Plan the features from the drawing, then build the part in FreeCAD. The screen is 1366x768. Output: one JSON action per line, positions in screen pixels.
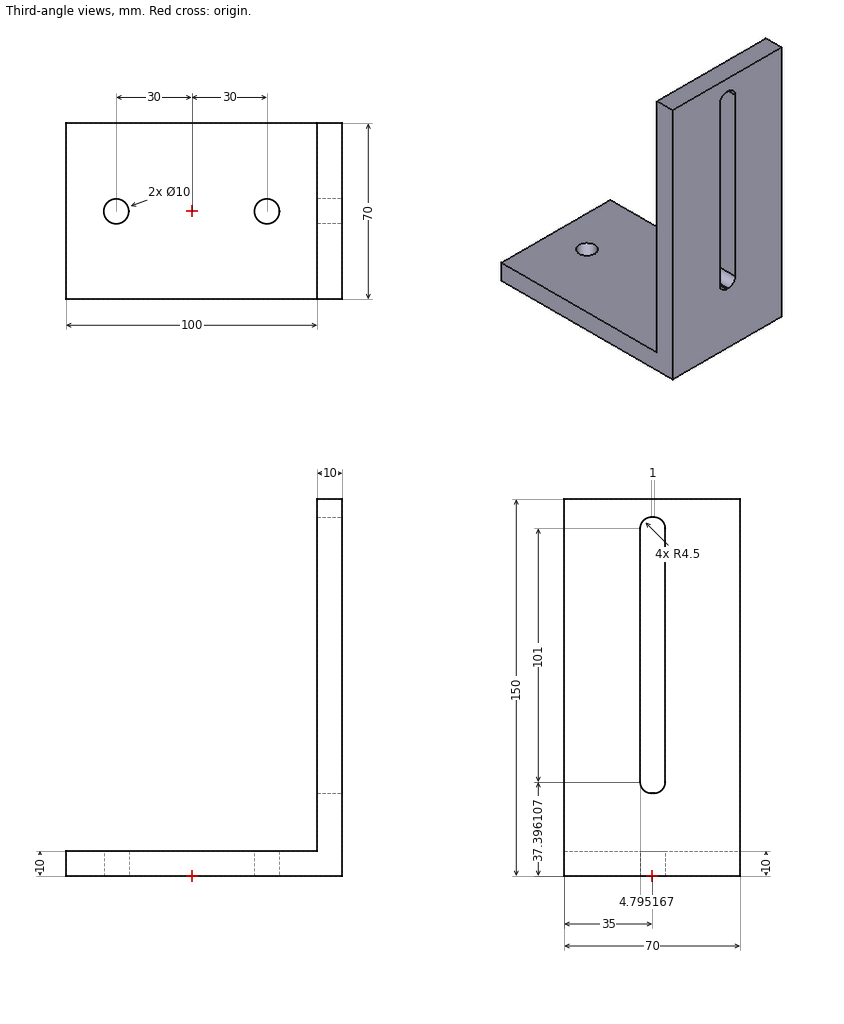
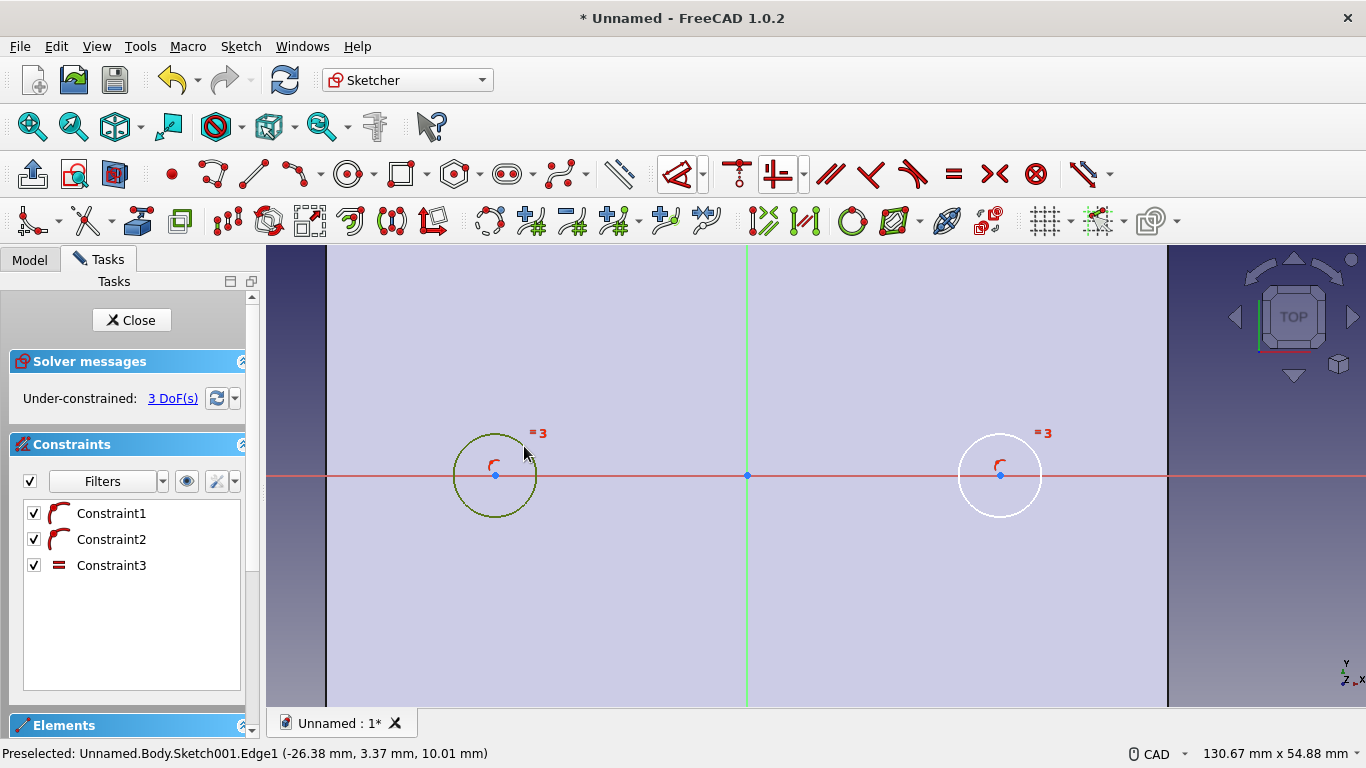
{"action": "left_click", "coordinate": [702, 174]}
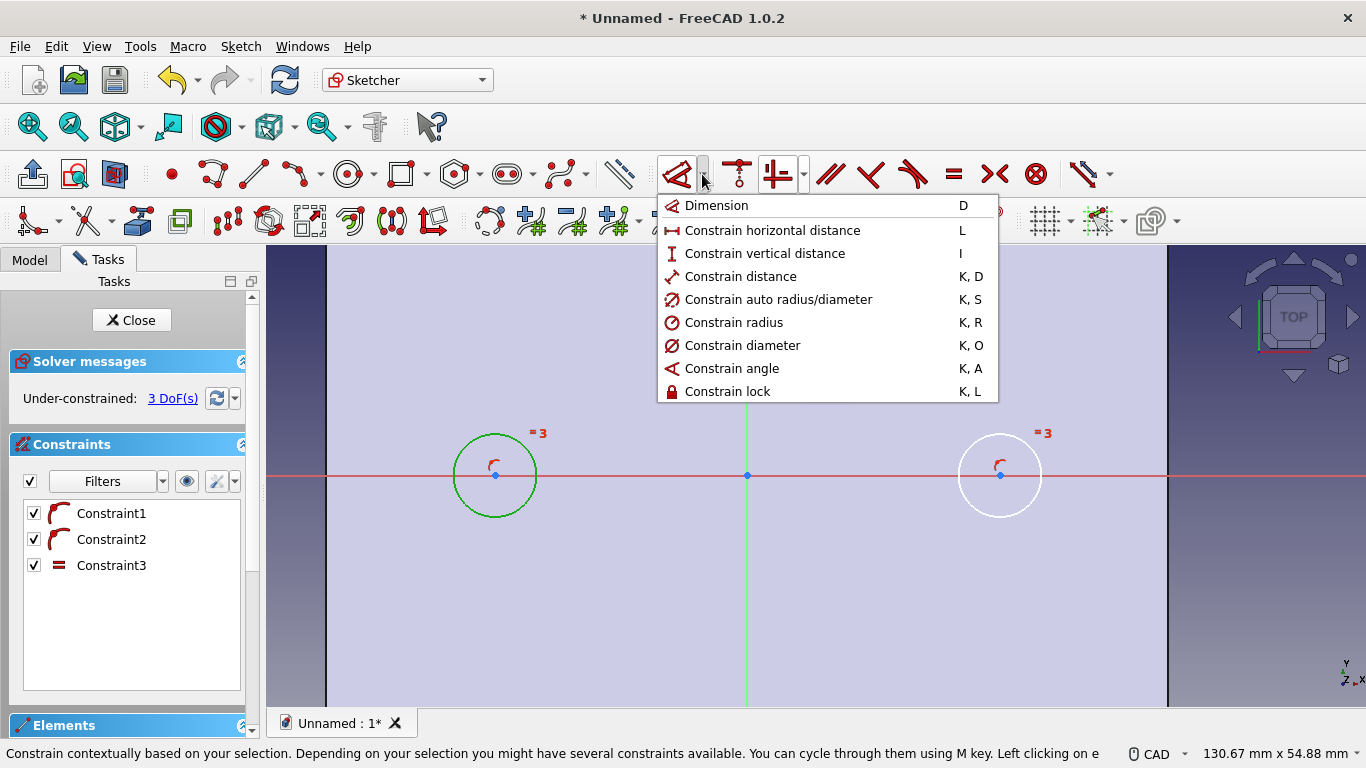
{"action": "left_click", "coordinate": [828, 346]}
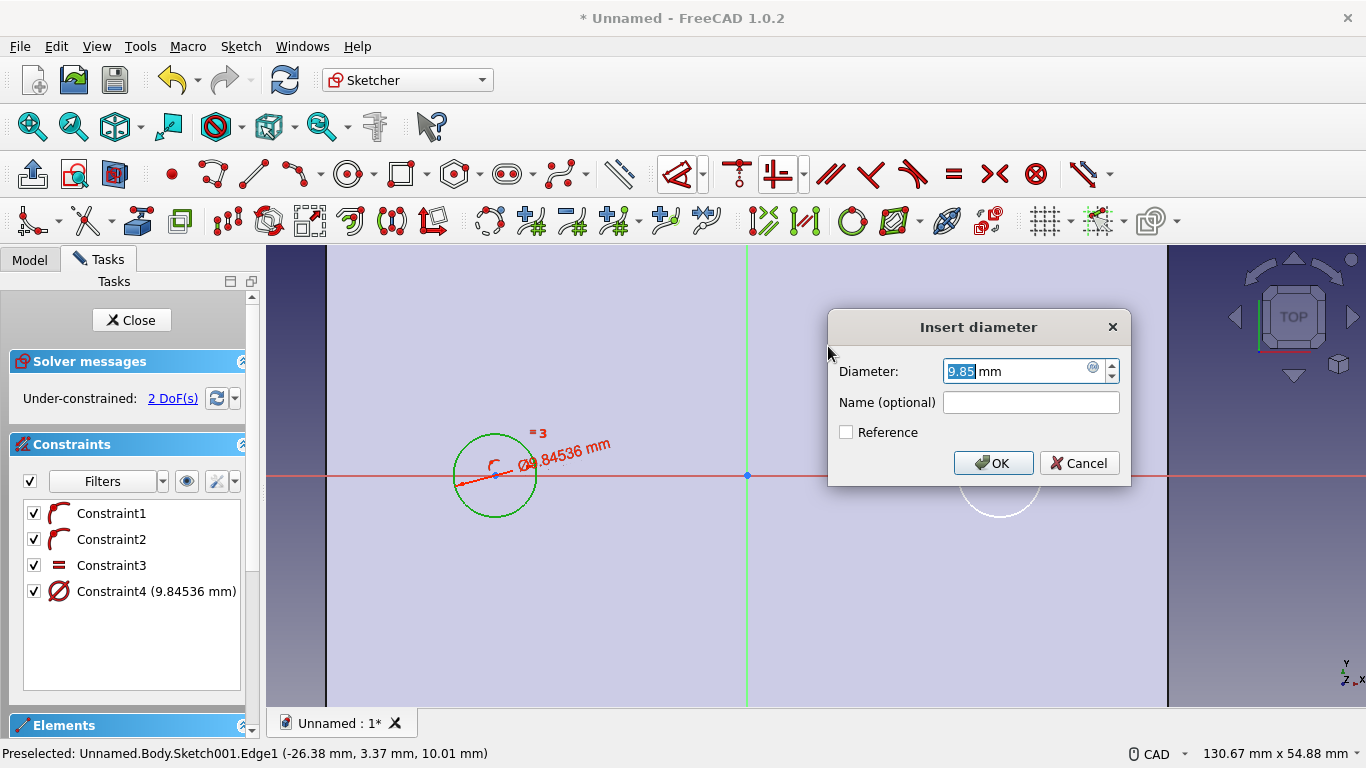
{"action": "type", "text": "10"}
{"action": "key", "text": "Return"}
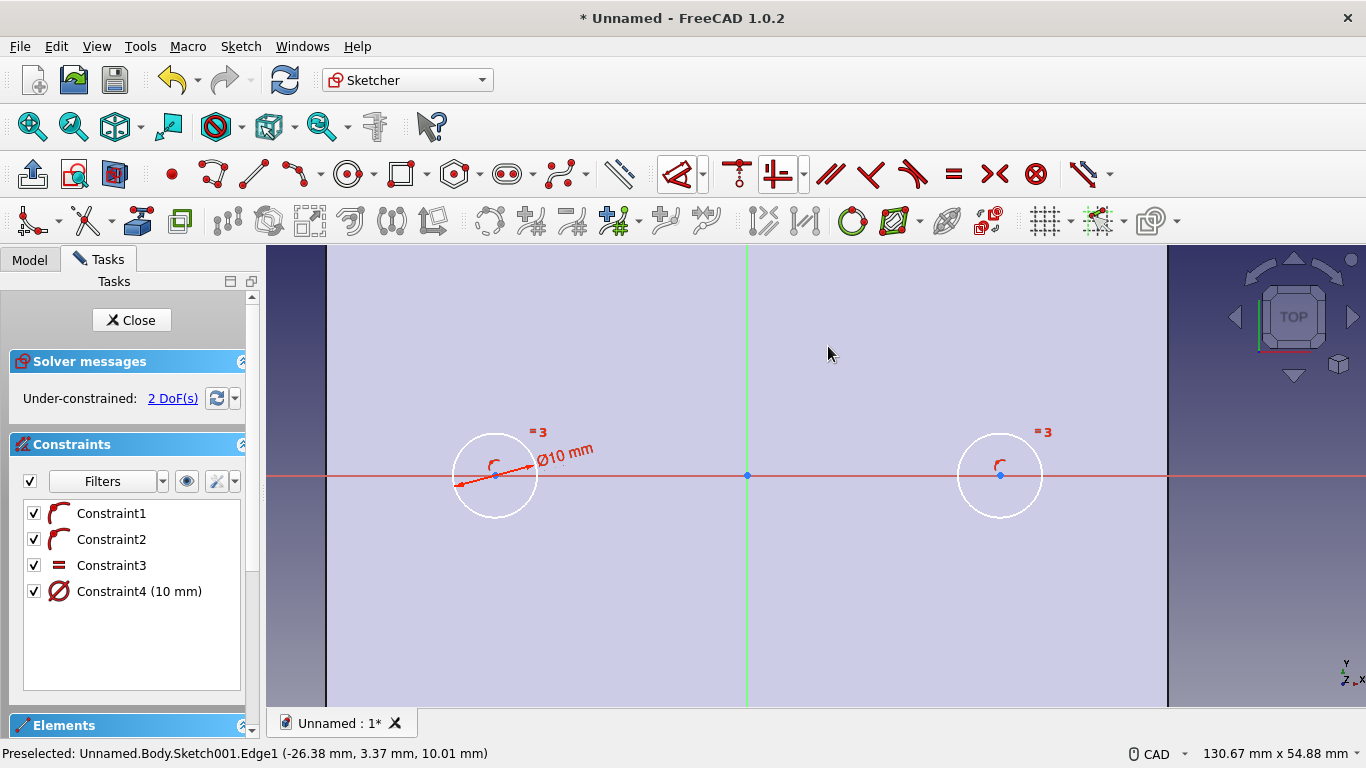
{"action": "left_click", "coordinate": [495, 476]}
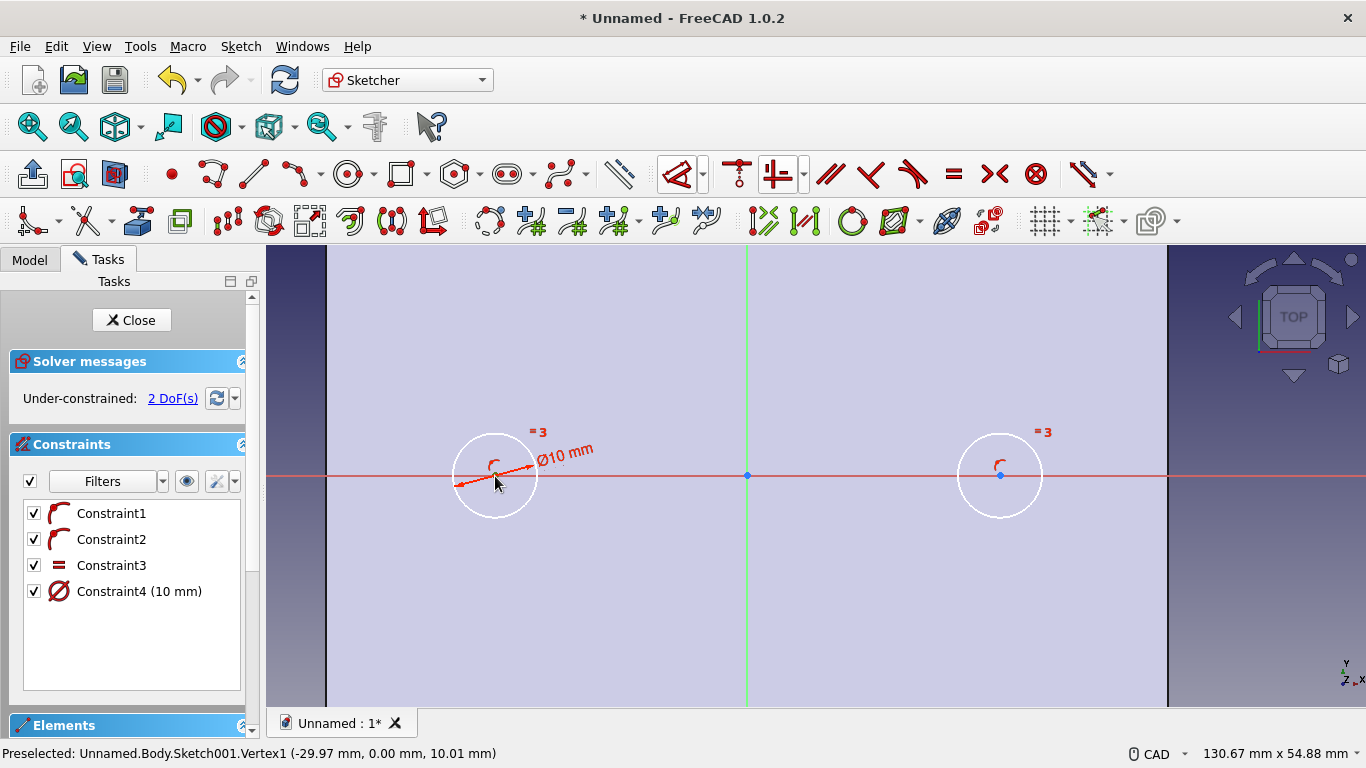
{"action": "left_click", "coordinate": [702, 174]}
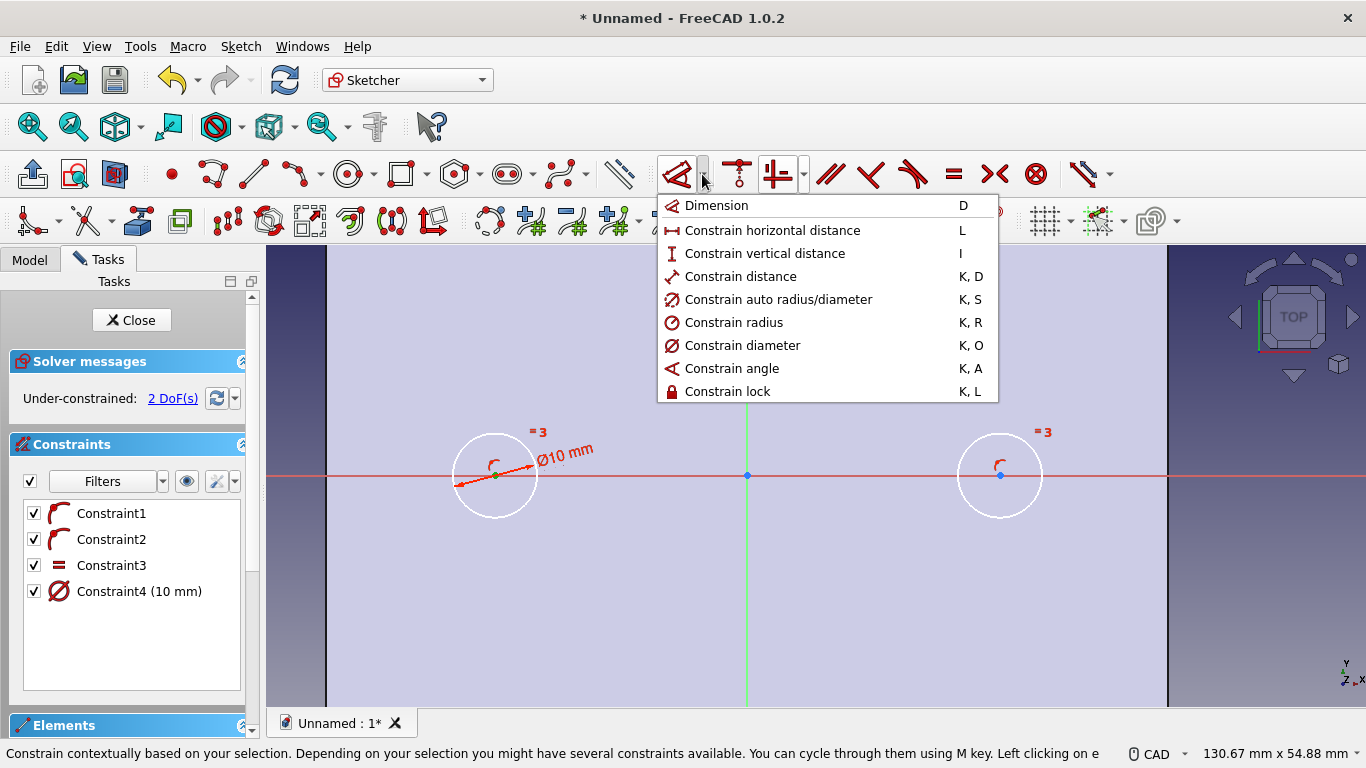
{"action": "left_click", "coordinate": [828, 230]}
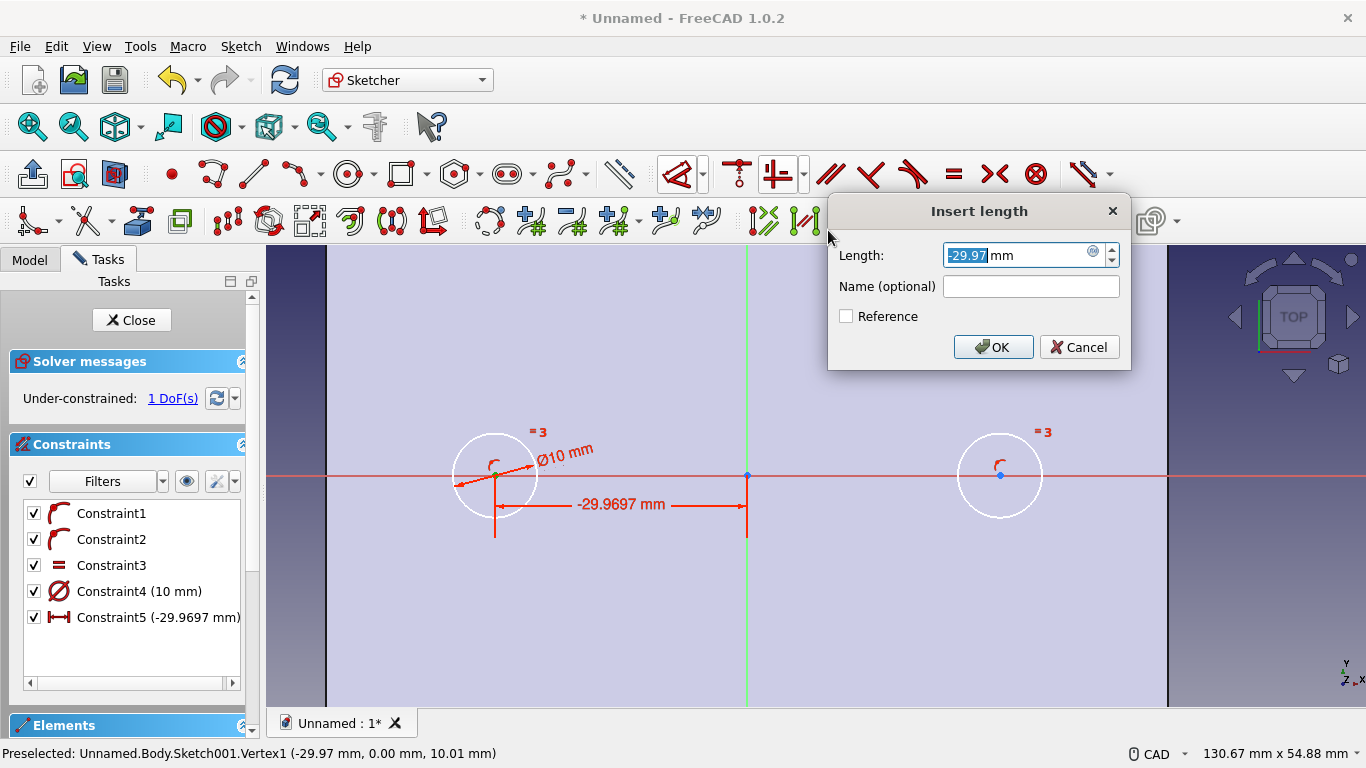
{"action": "type", "text": "-30"}
{"action": "key", "text": "Return"}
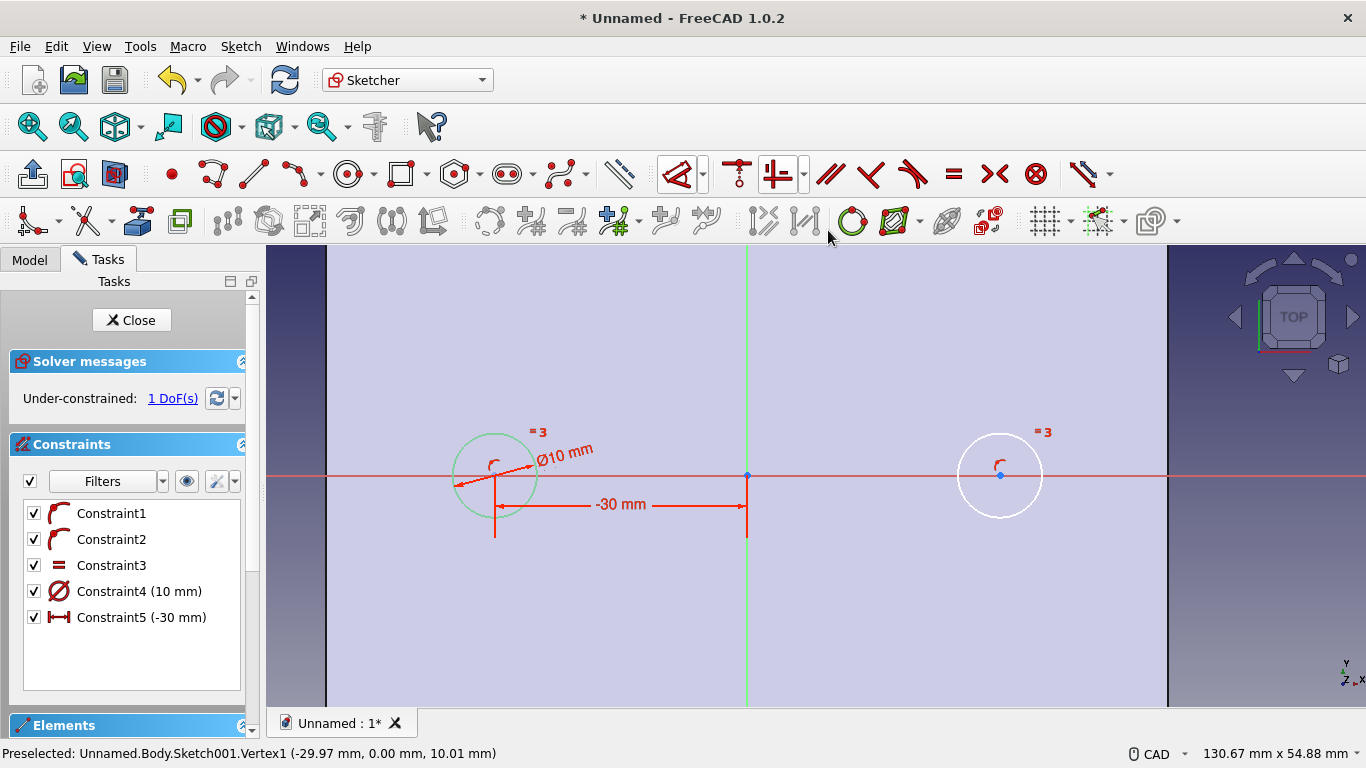
{"action": "left_click", "coordinate": [1000, 476]}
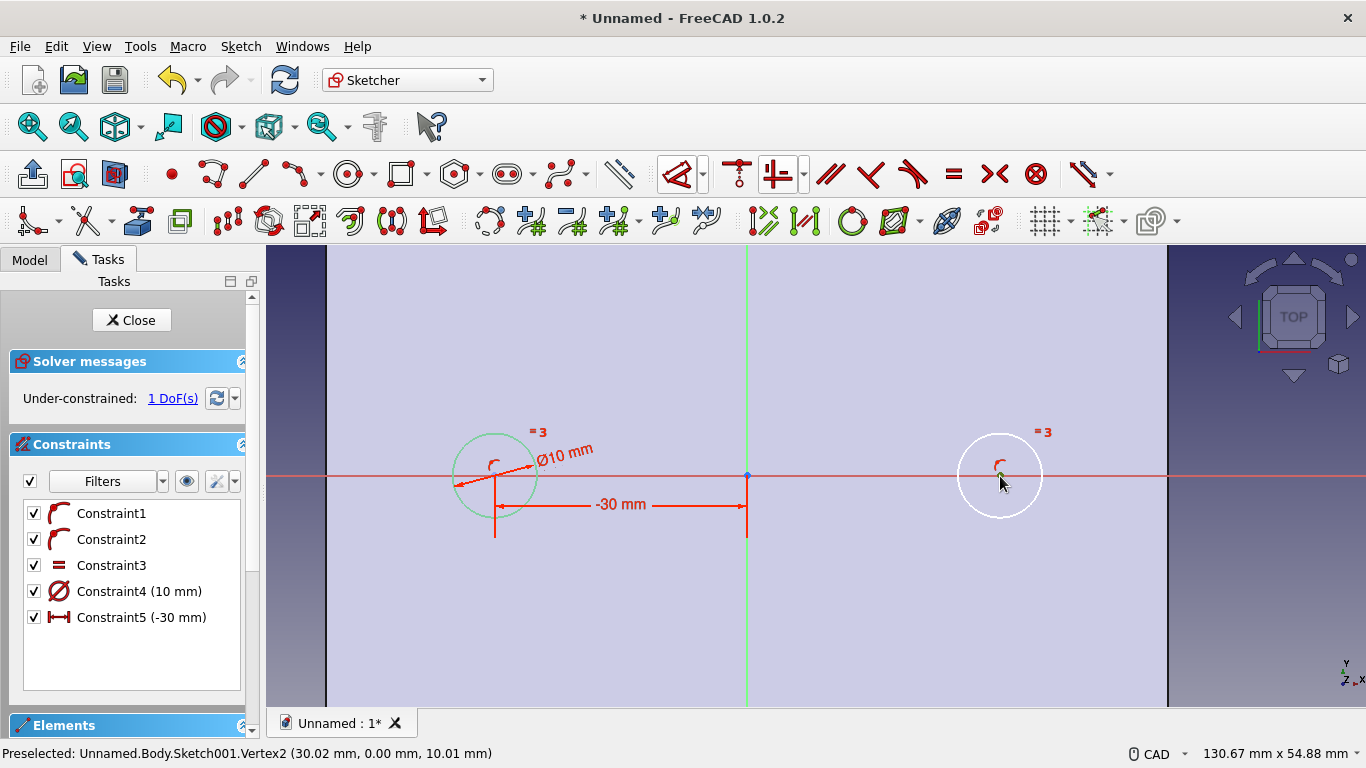
{"action": "left_click", "coordinate": [702, 174]}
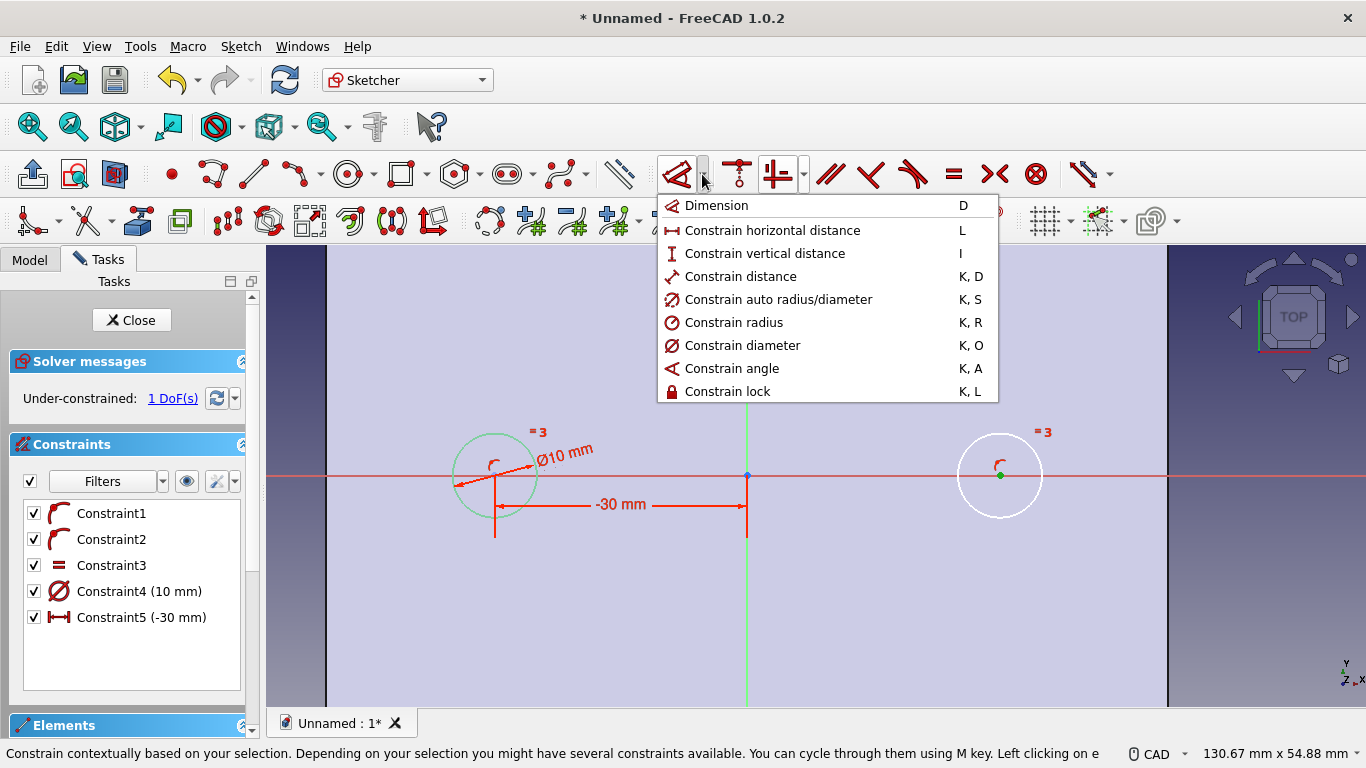
{"action": "left_click", "coordinate": [828, 230]}